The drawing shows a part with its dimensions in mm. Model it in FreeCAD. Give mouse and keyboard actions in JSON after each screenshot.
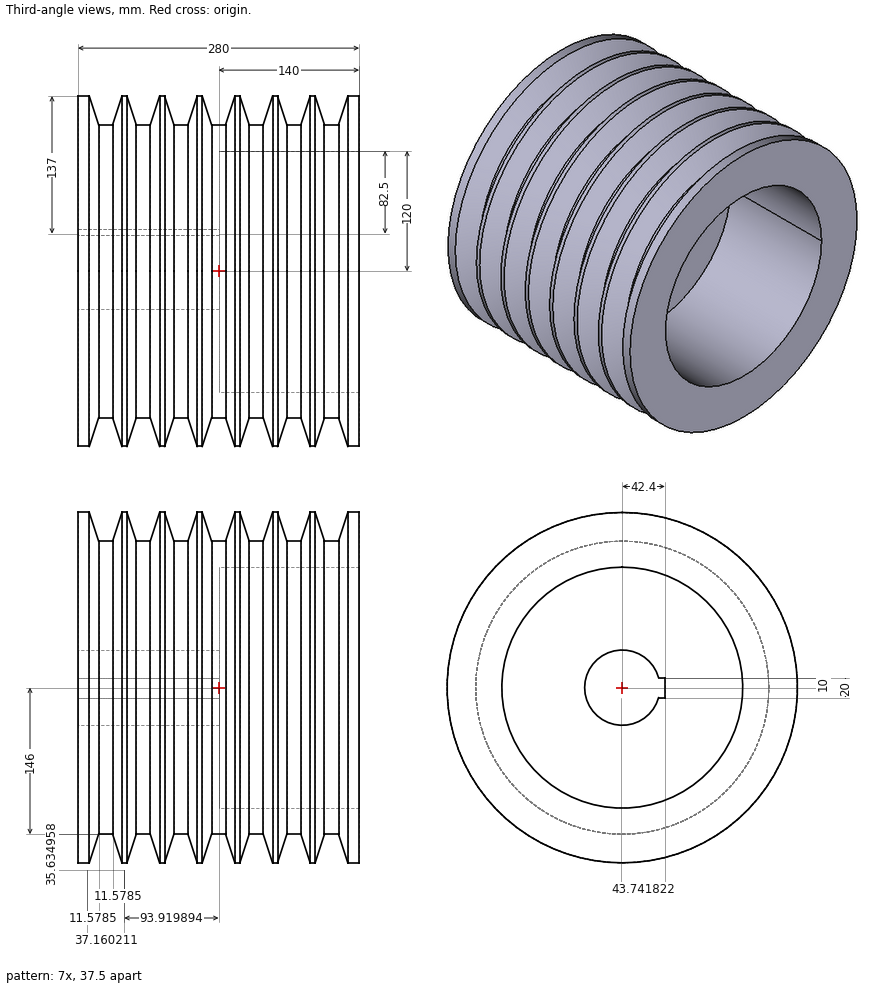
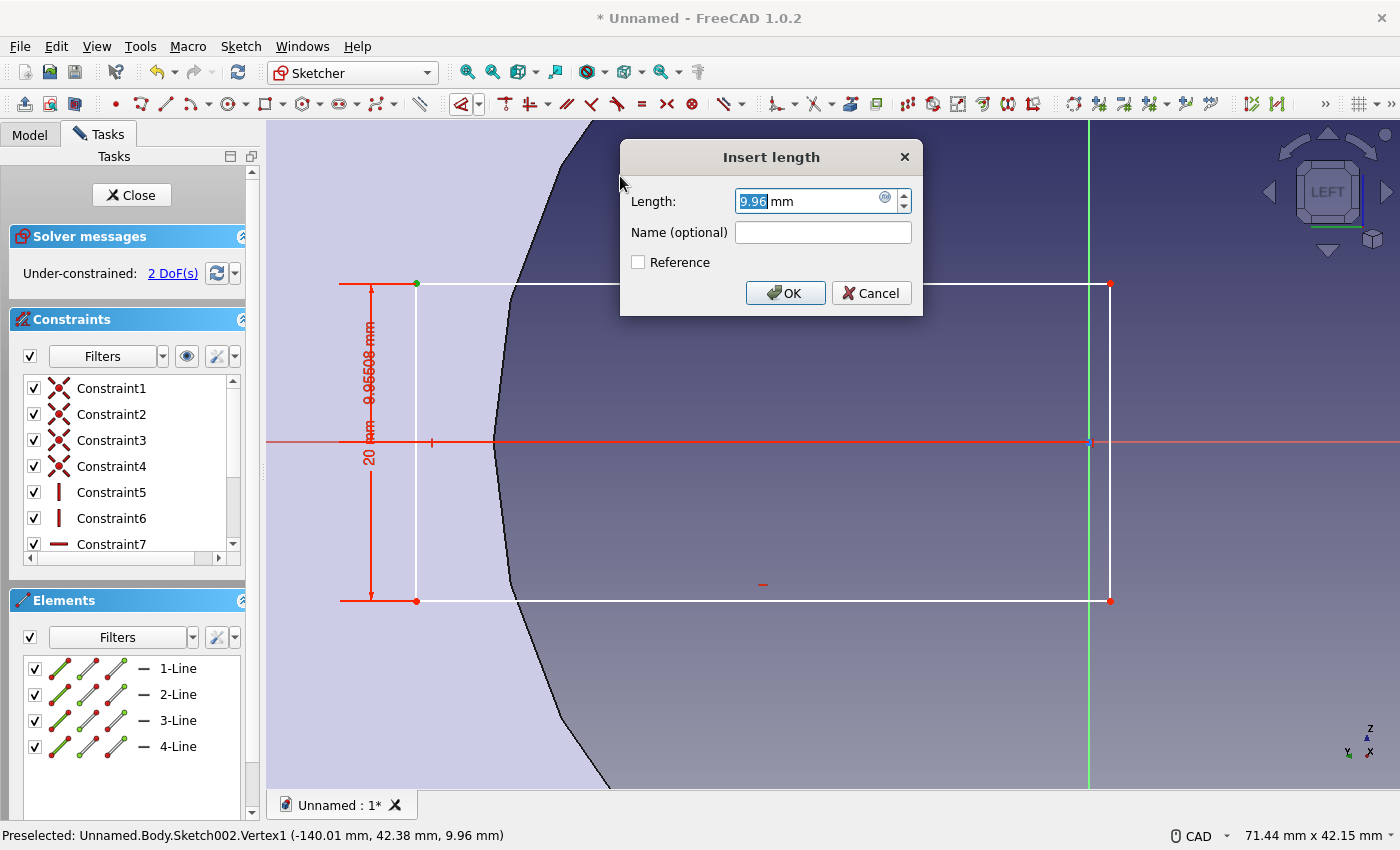
{"action": "type", "text": "10"}
{"action": "key", "text": "Return"}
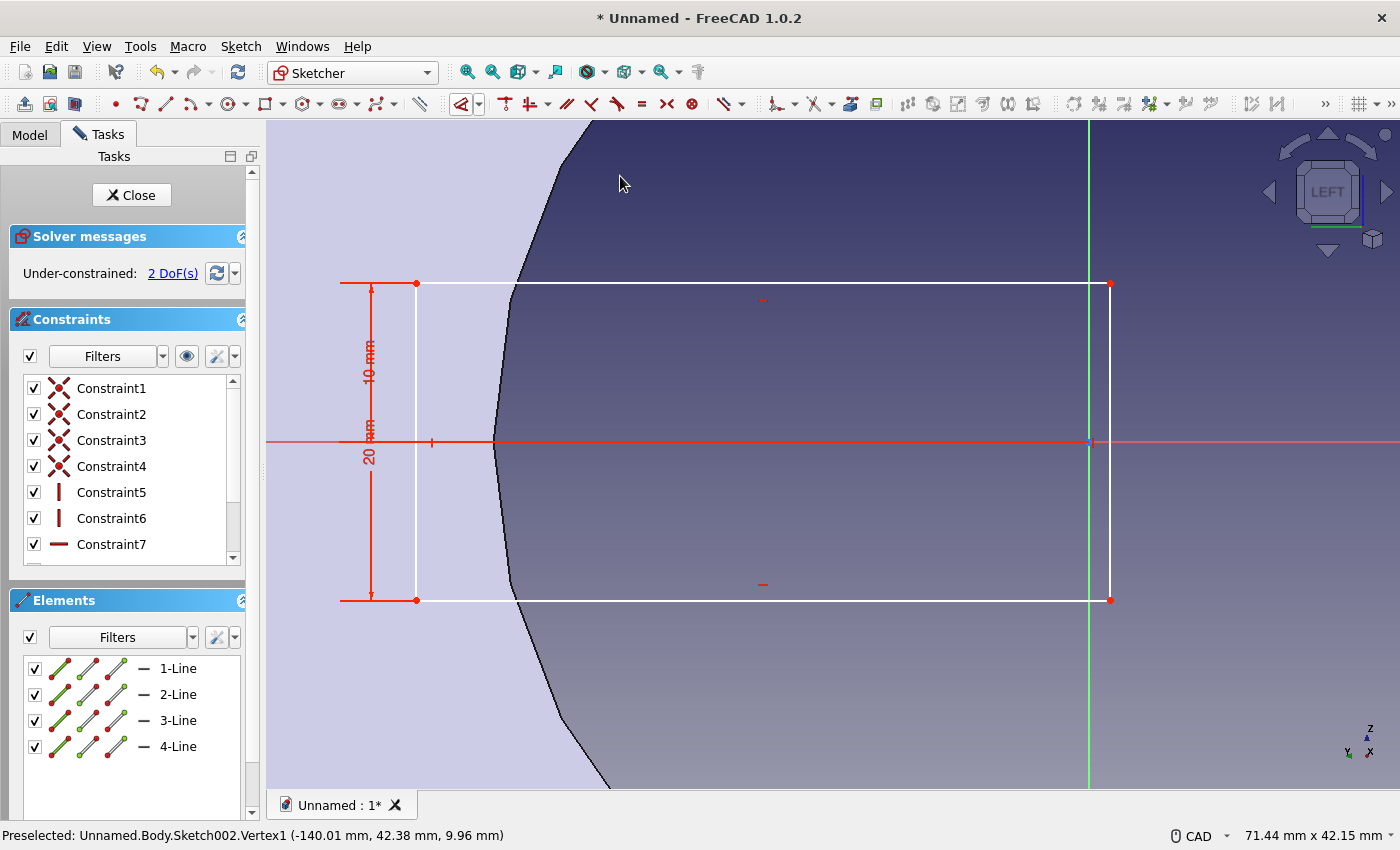
{"action": "left_click", "coordinate": [416, 283]}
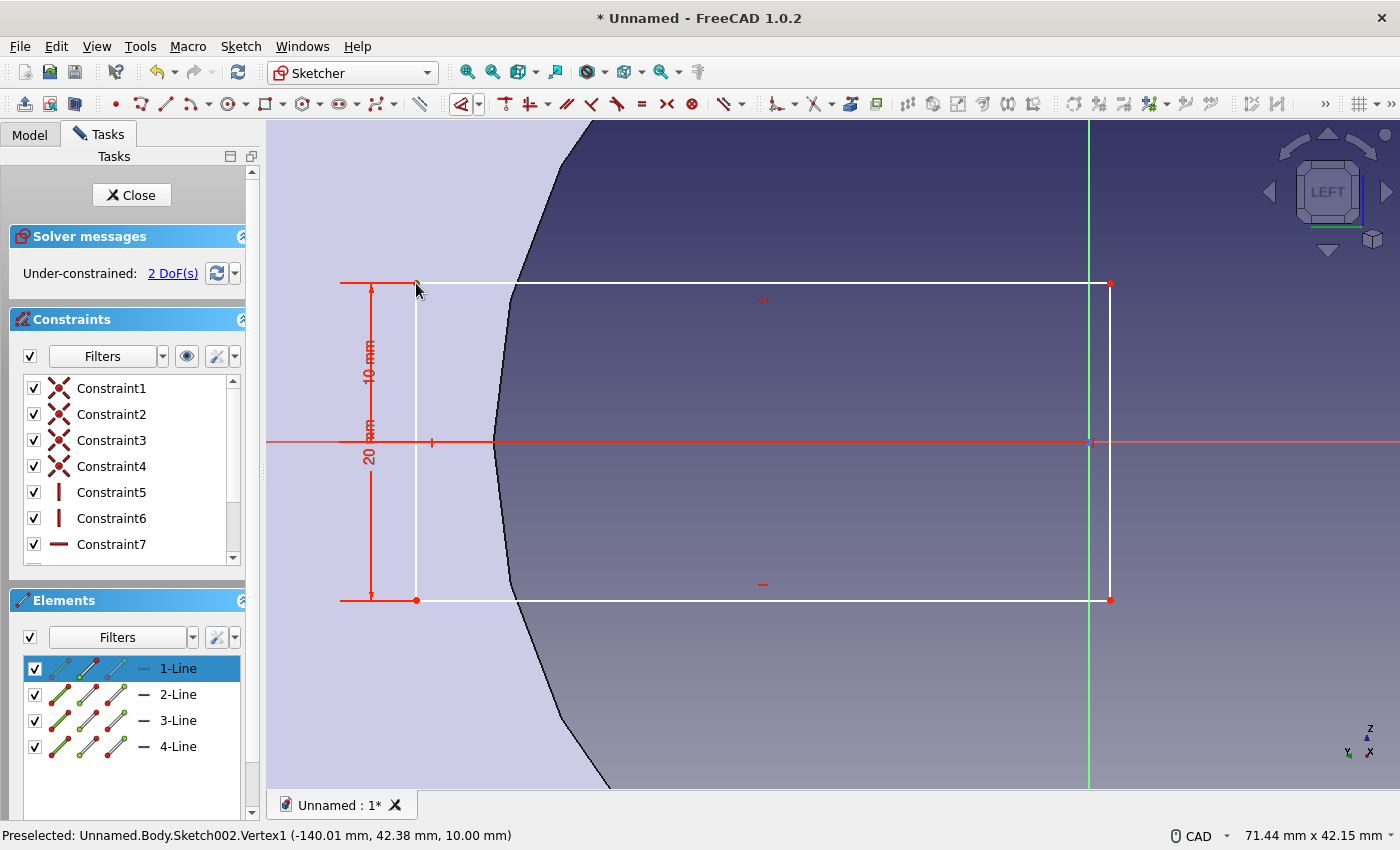
{"action": "left_click", "coordinate": [478, 104]}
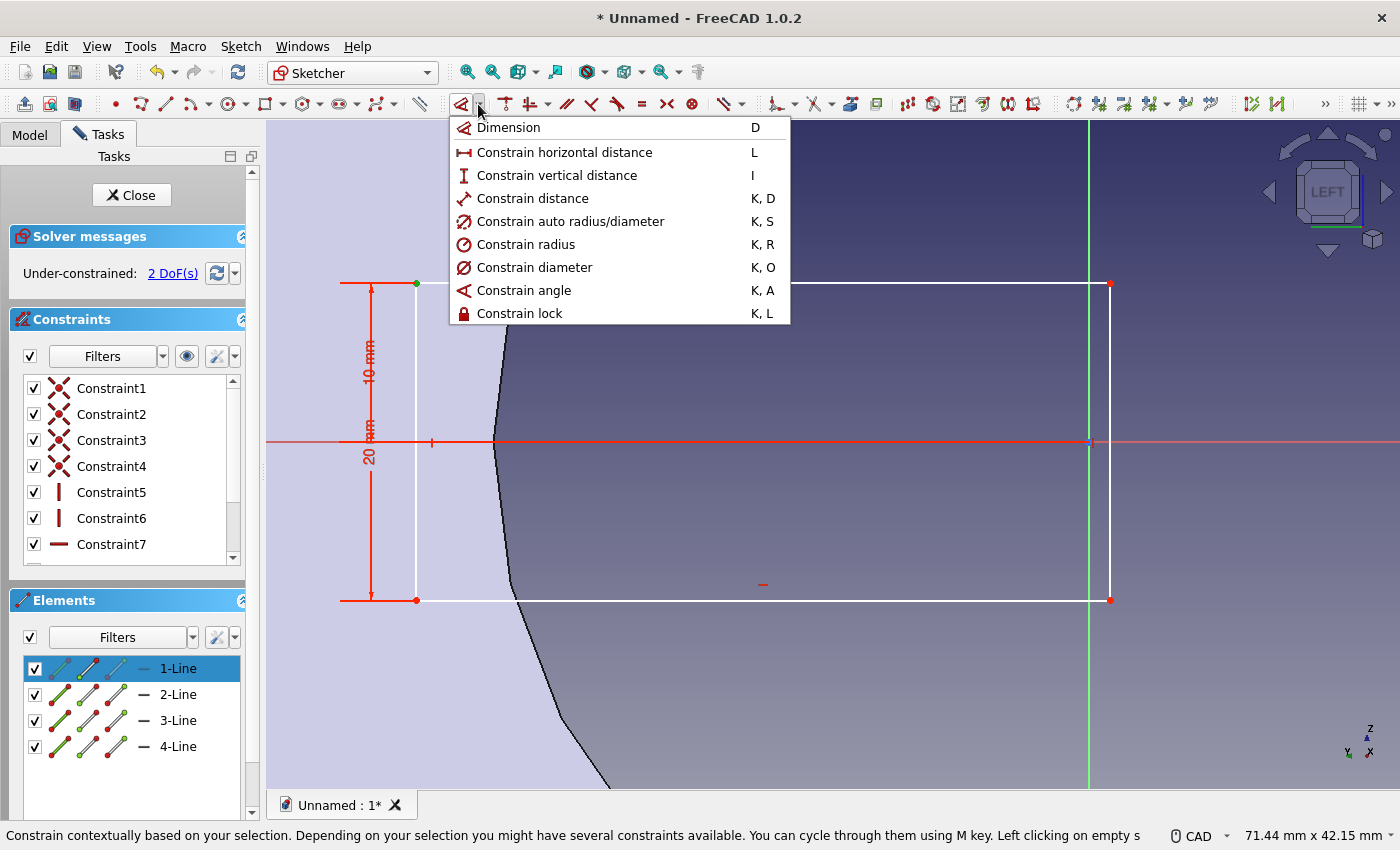
{"action": "left_click", "coordinate": [620, 152]}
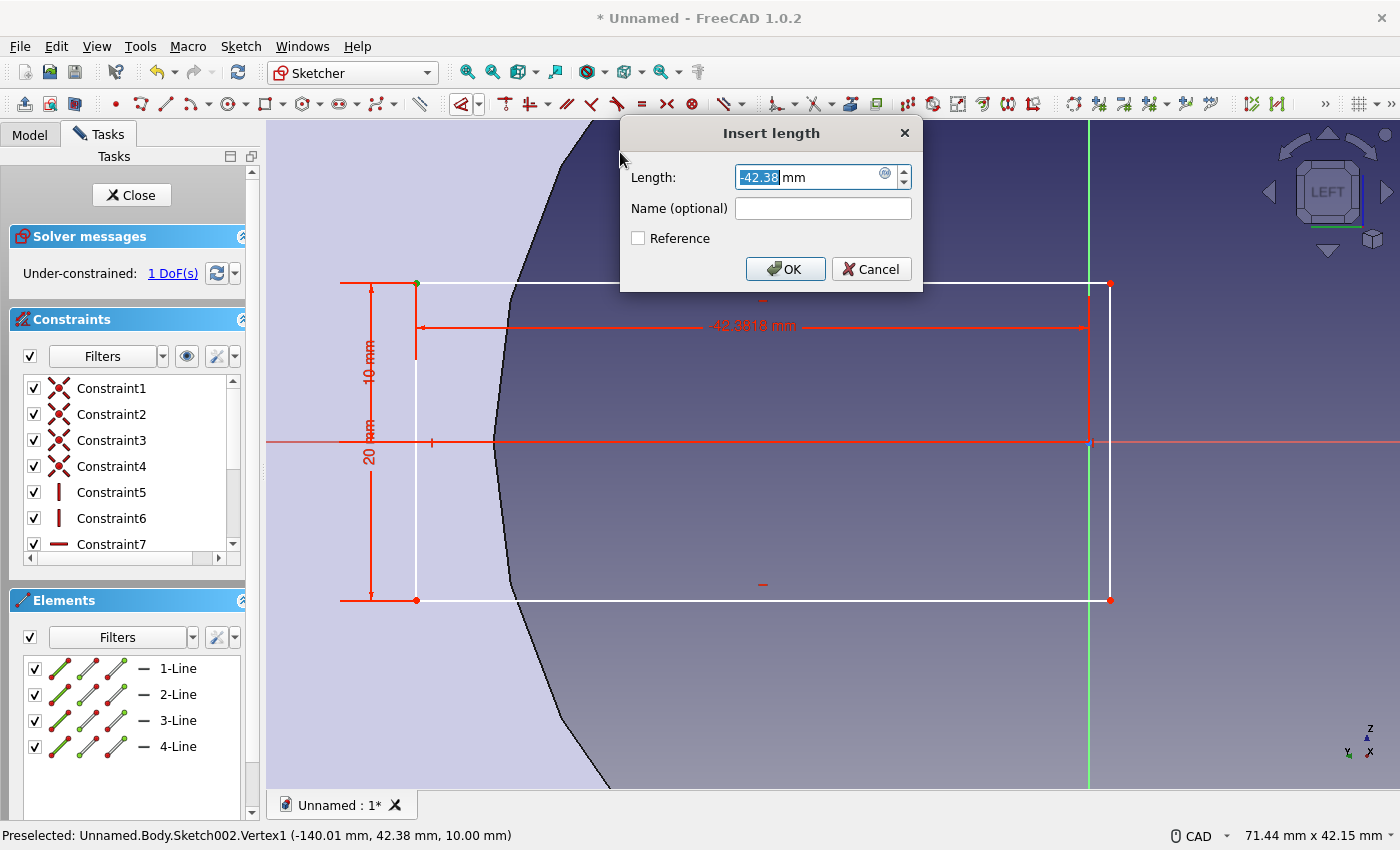
{"action": "type", "text": "-42.4"}
{"action": "key", "text": "Return"}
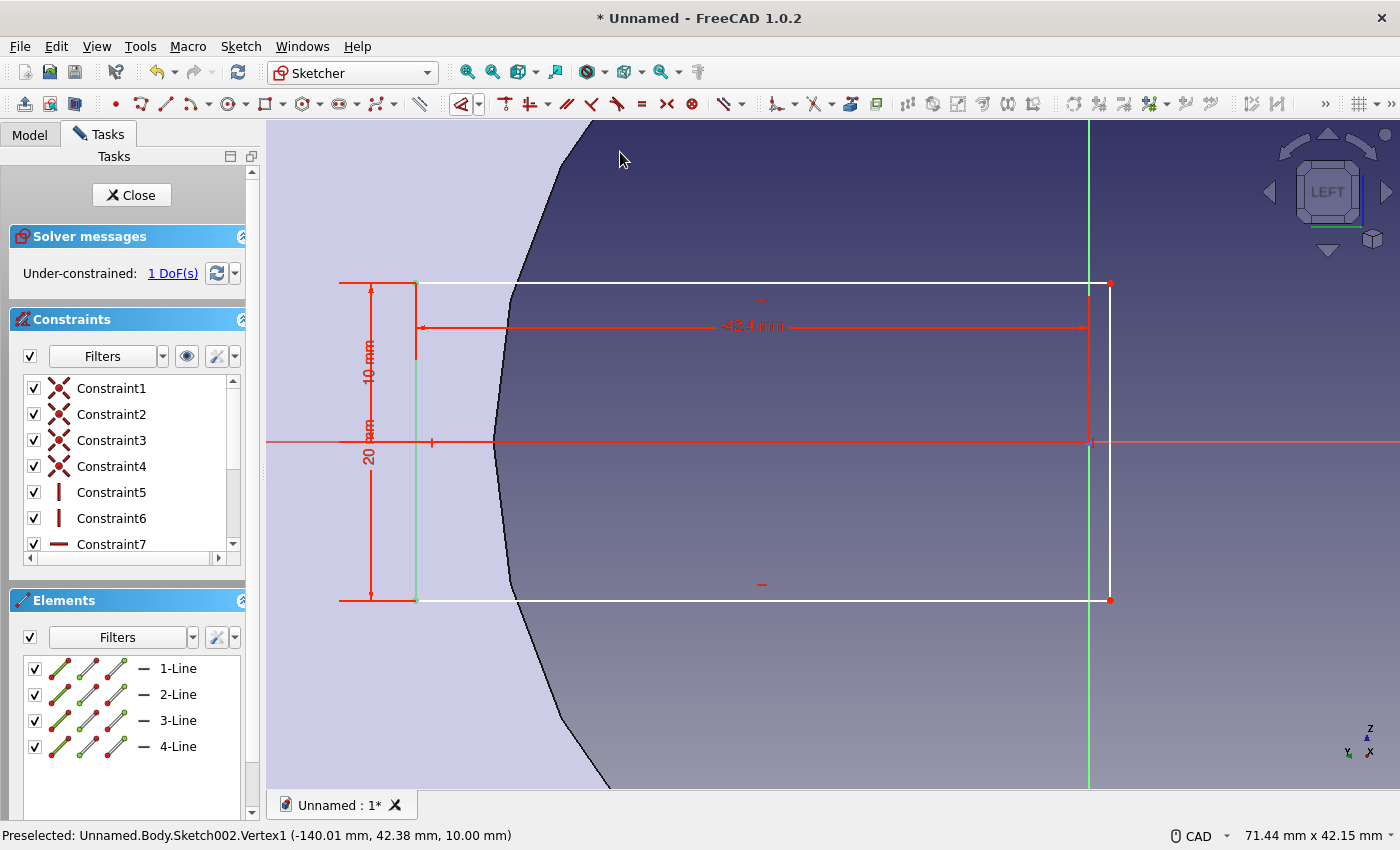
{"action": "left_click", "coordinate": [624, 601]}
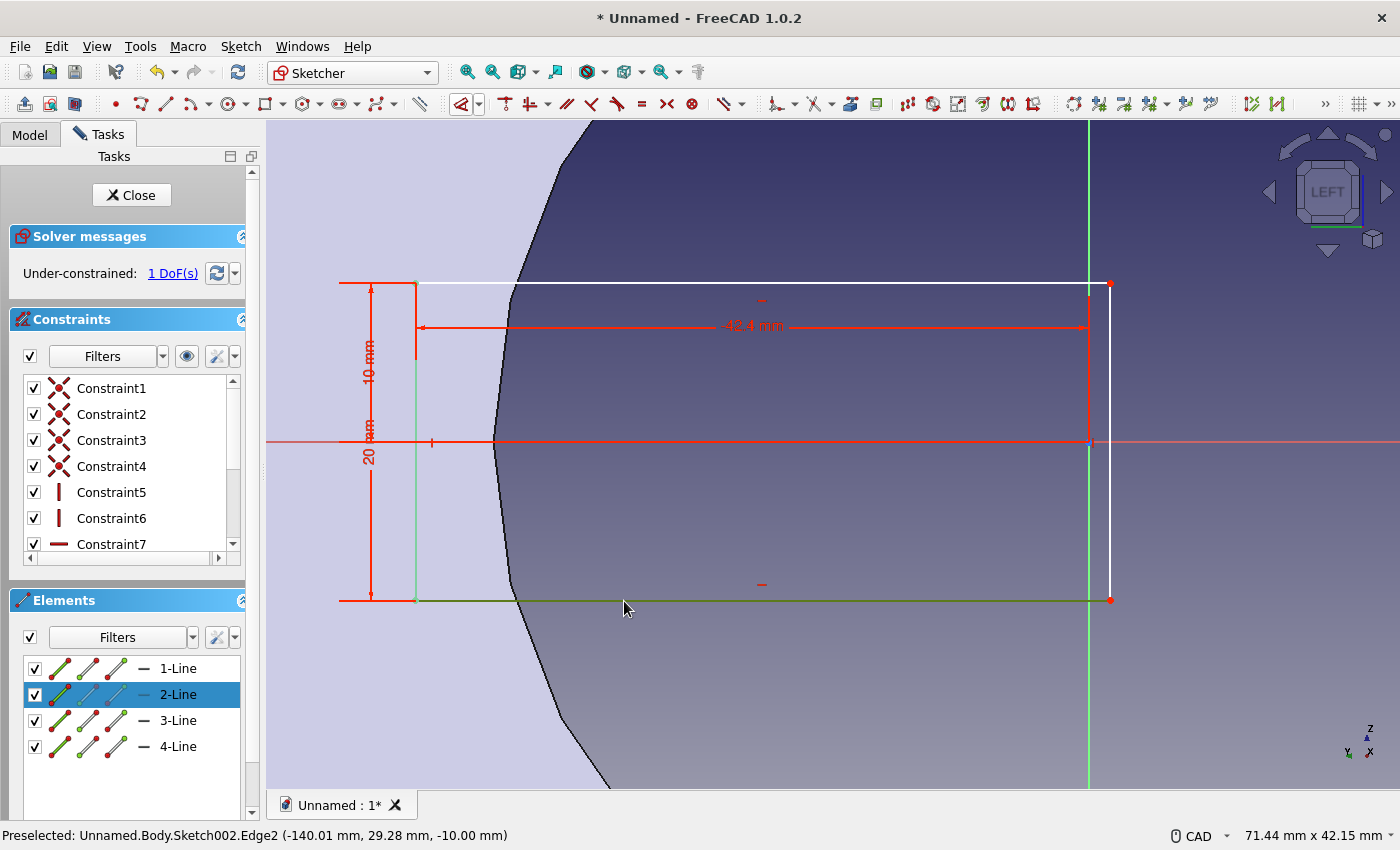
{"action": "key", "text": "l"}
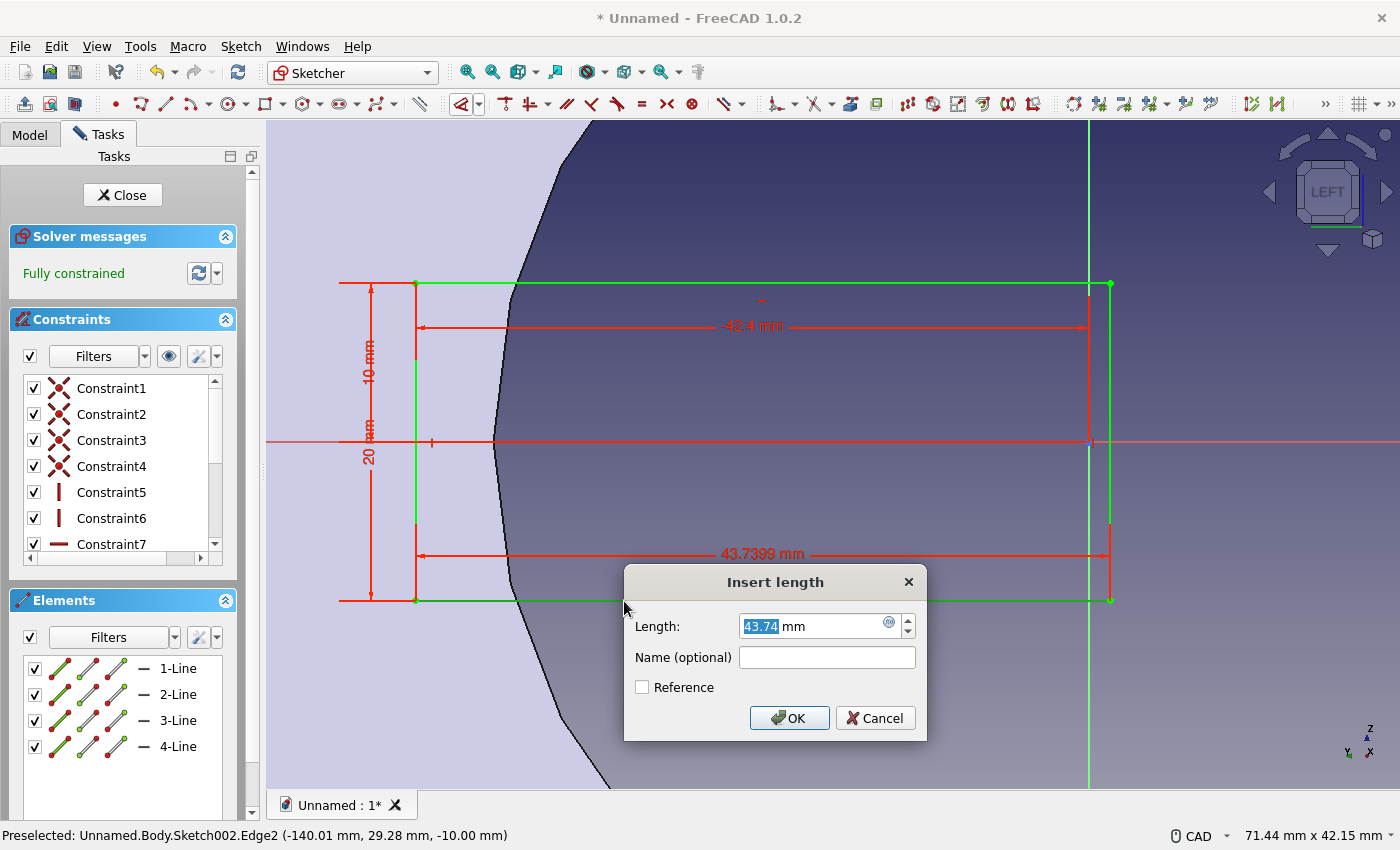
{"action": "type", "text": "43.741822"}
{"action": "key", "text": "Return"}